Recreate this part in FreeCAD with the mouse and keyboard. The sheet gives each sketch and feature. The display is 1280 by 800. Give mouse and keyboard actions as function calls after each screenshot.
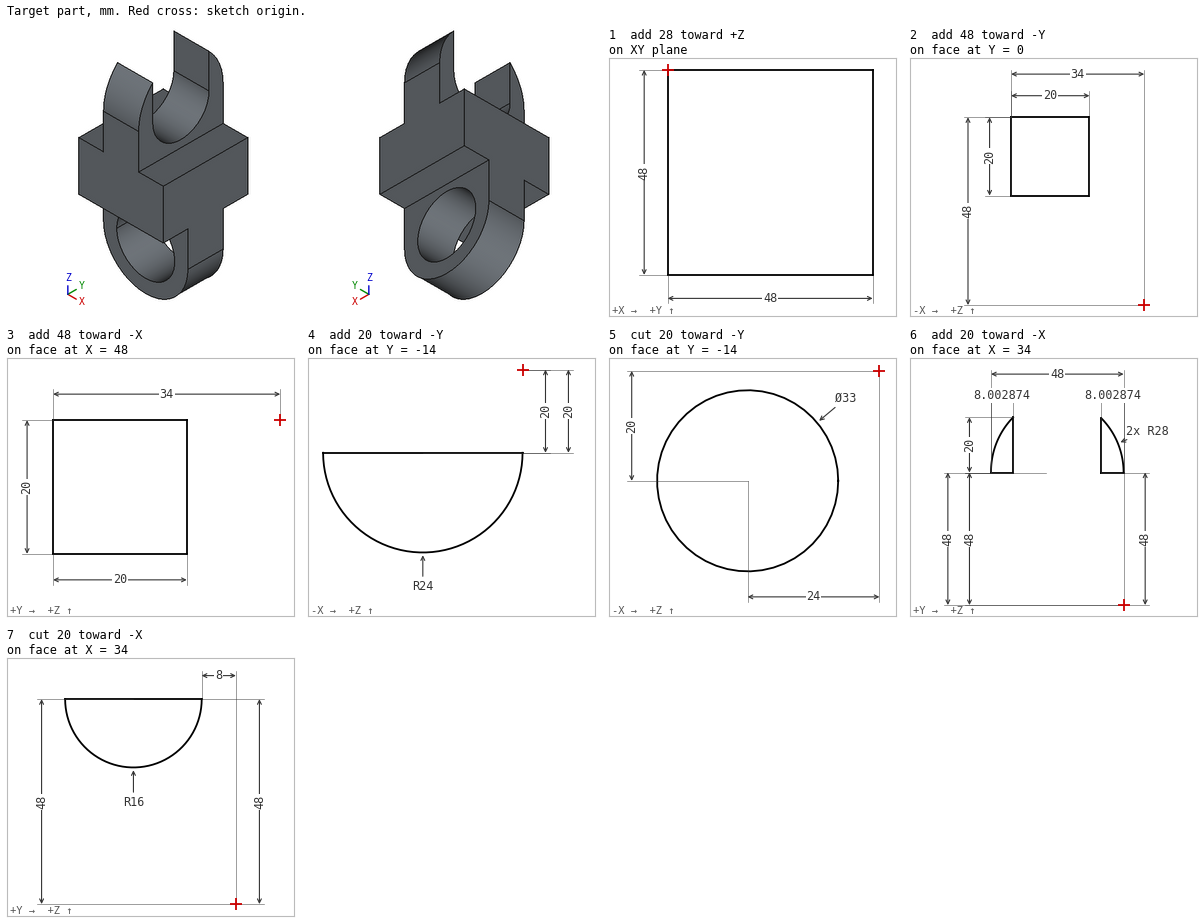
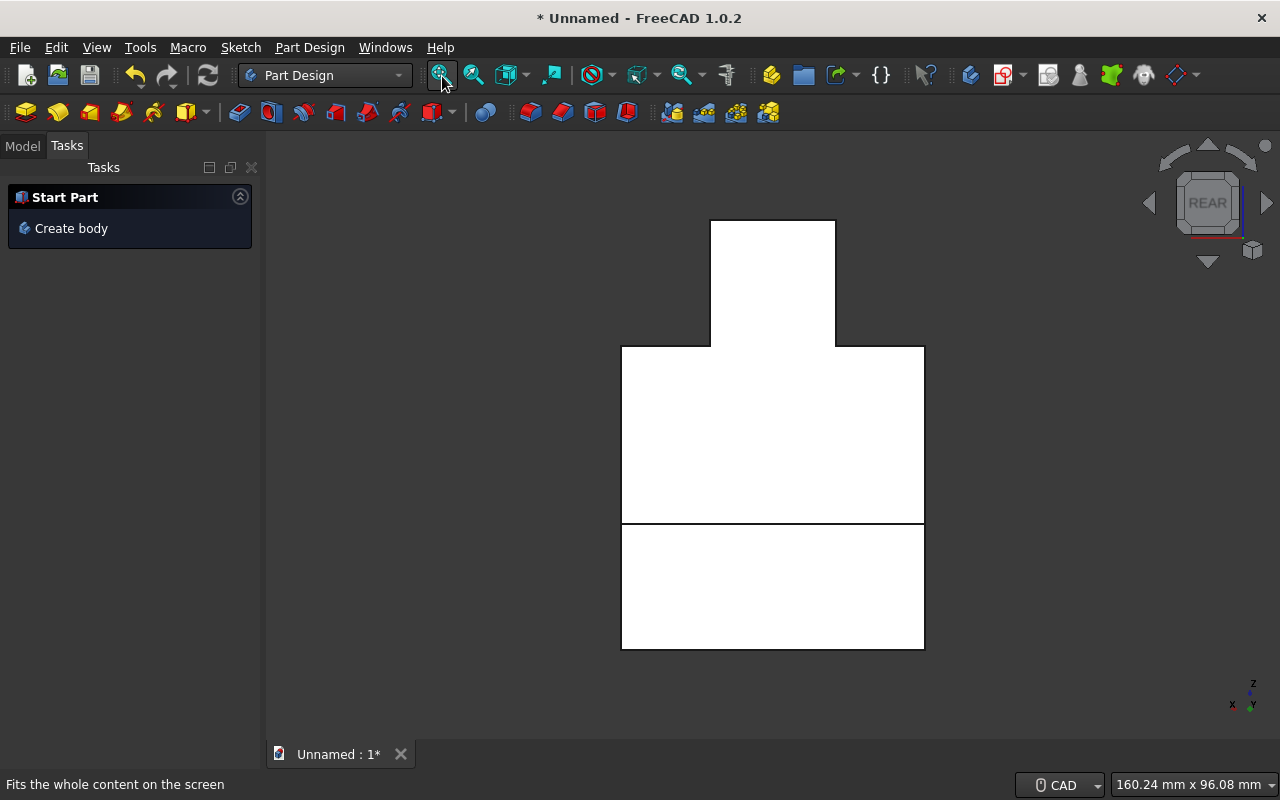
click(686, 586)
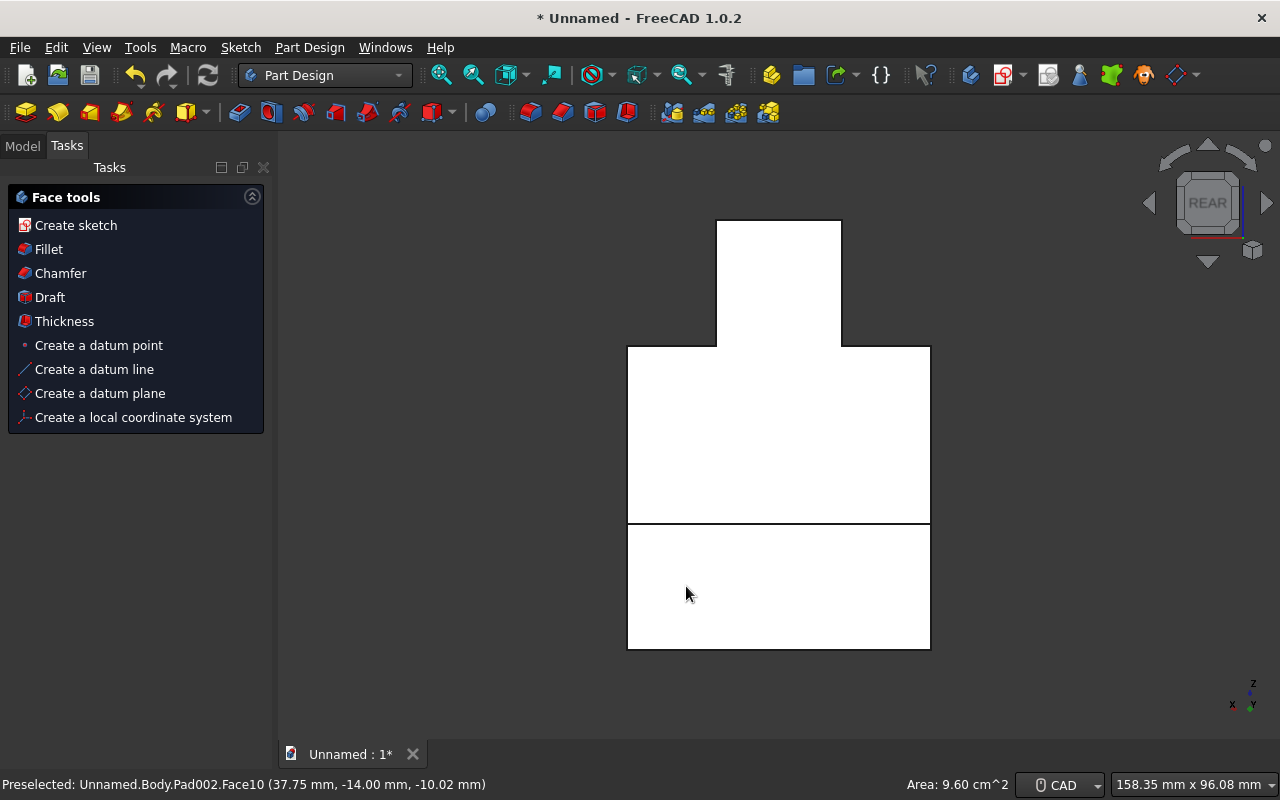
click(1004, 76)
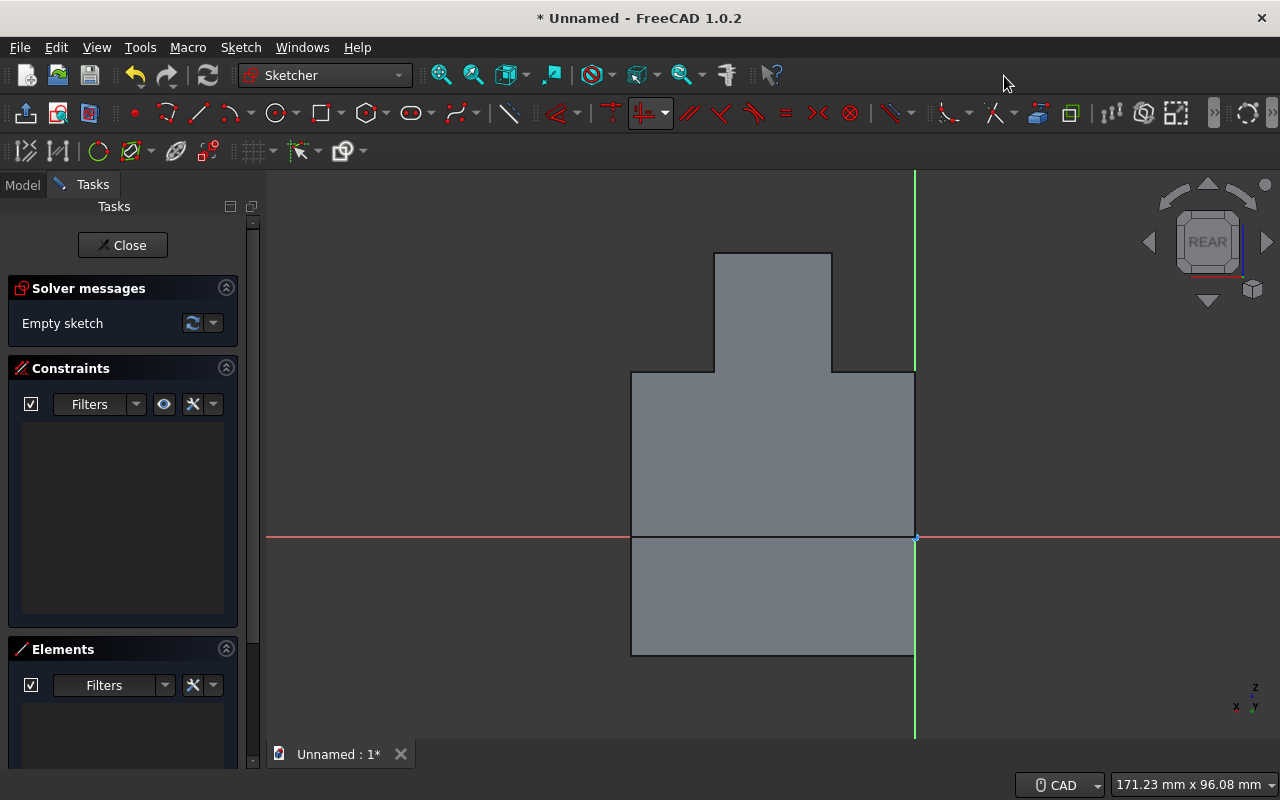
key(q)
key(s)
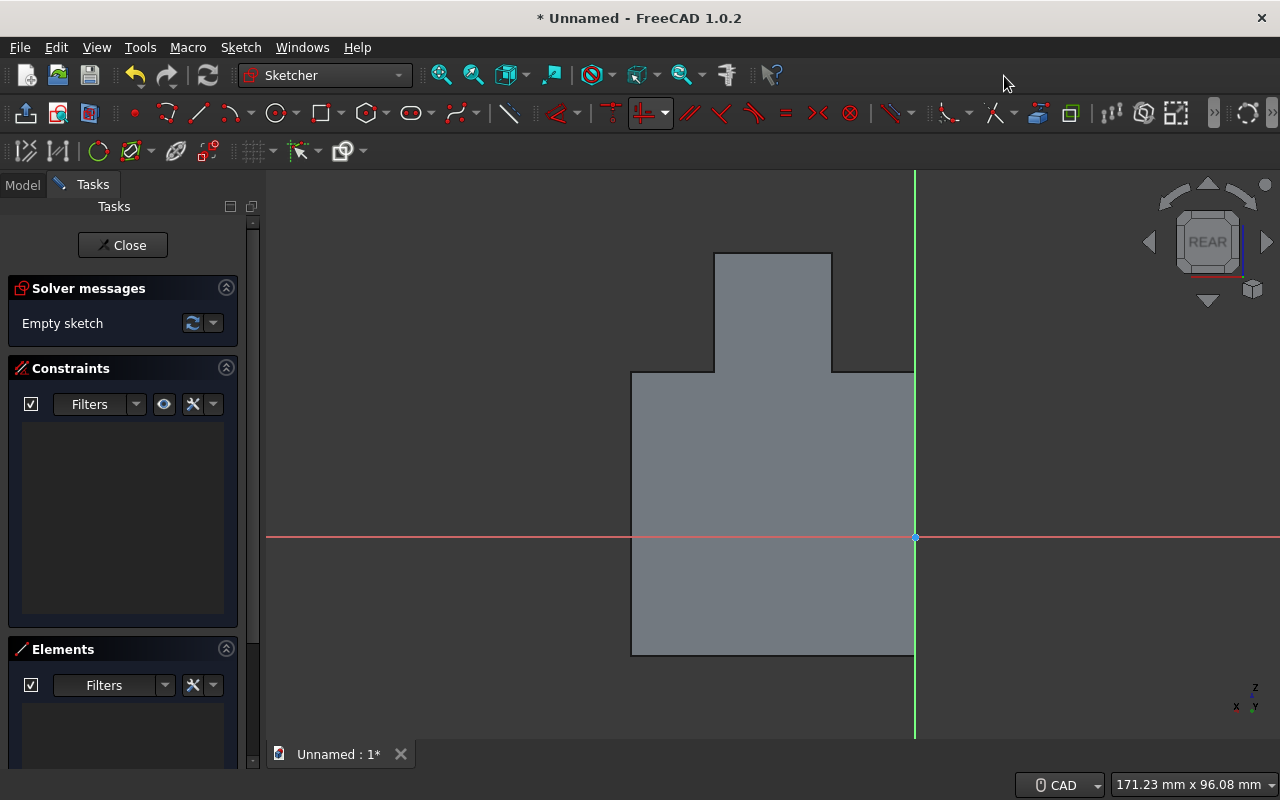
scroll(704, 454, down, 5)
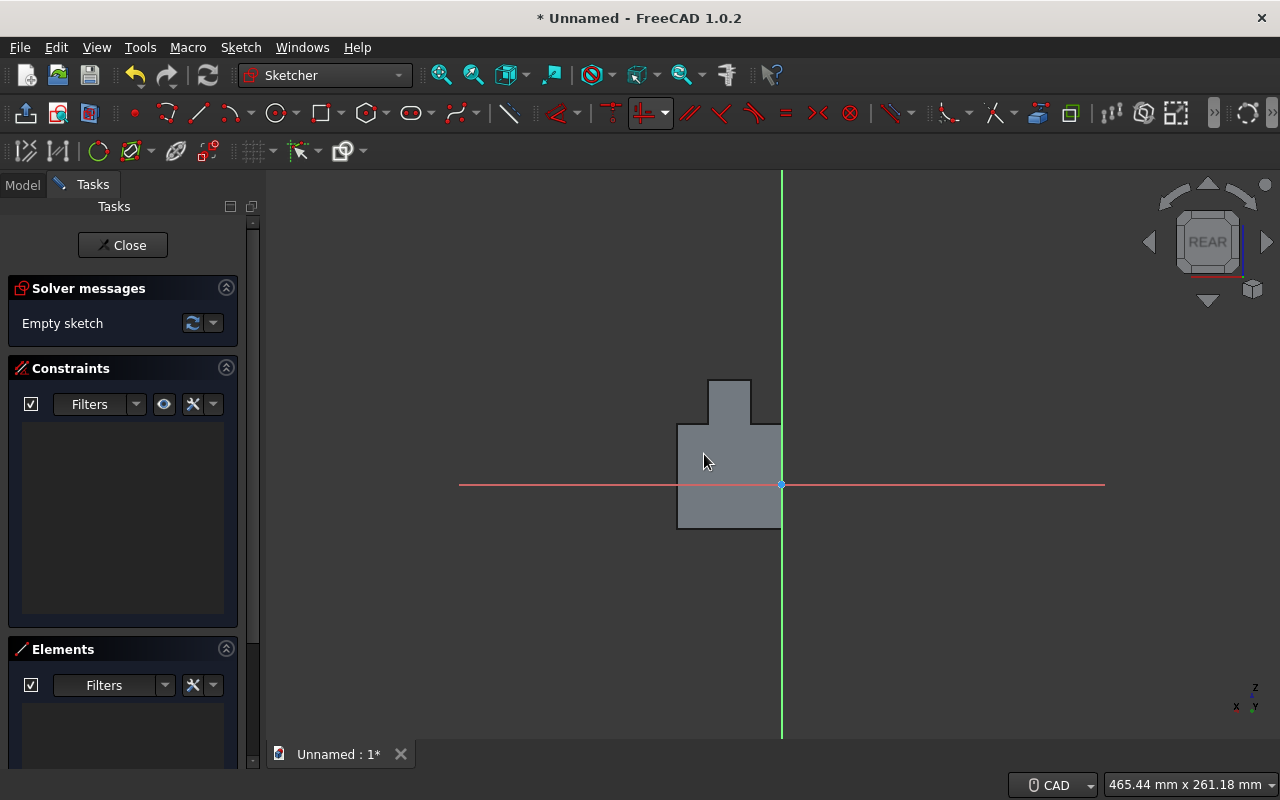
scroll(738, 559, up, 7)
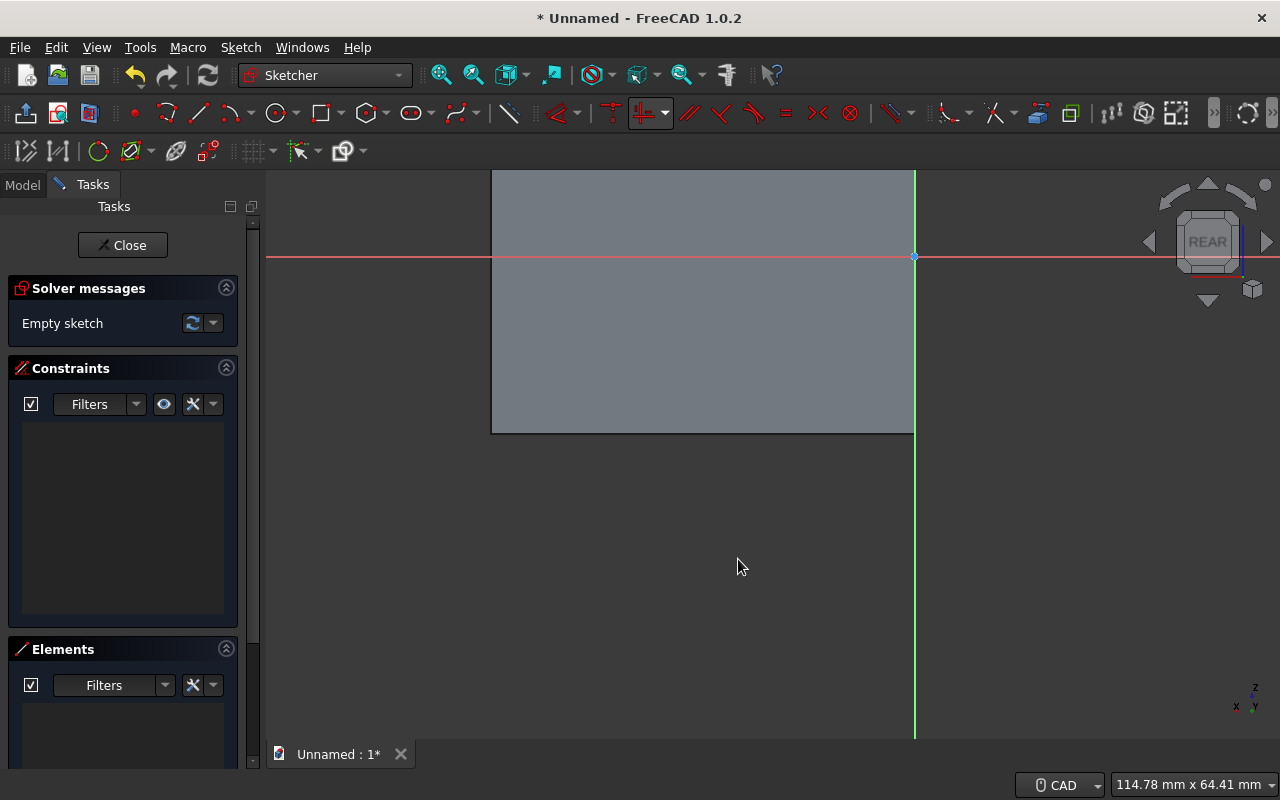
click(200, 114)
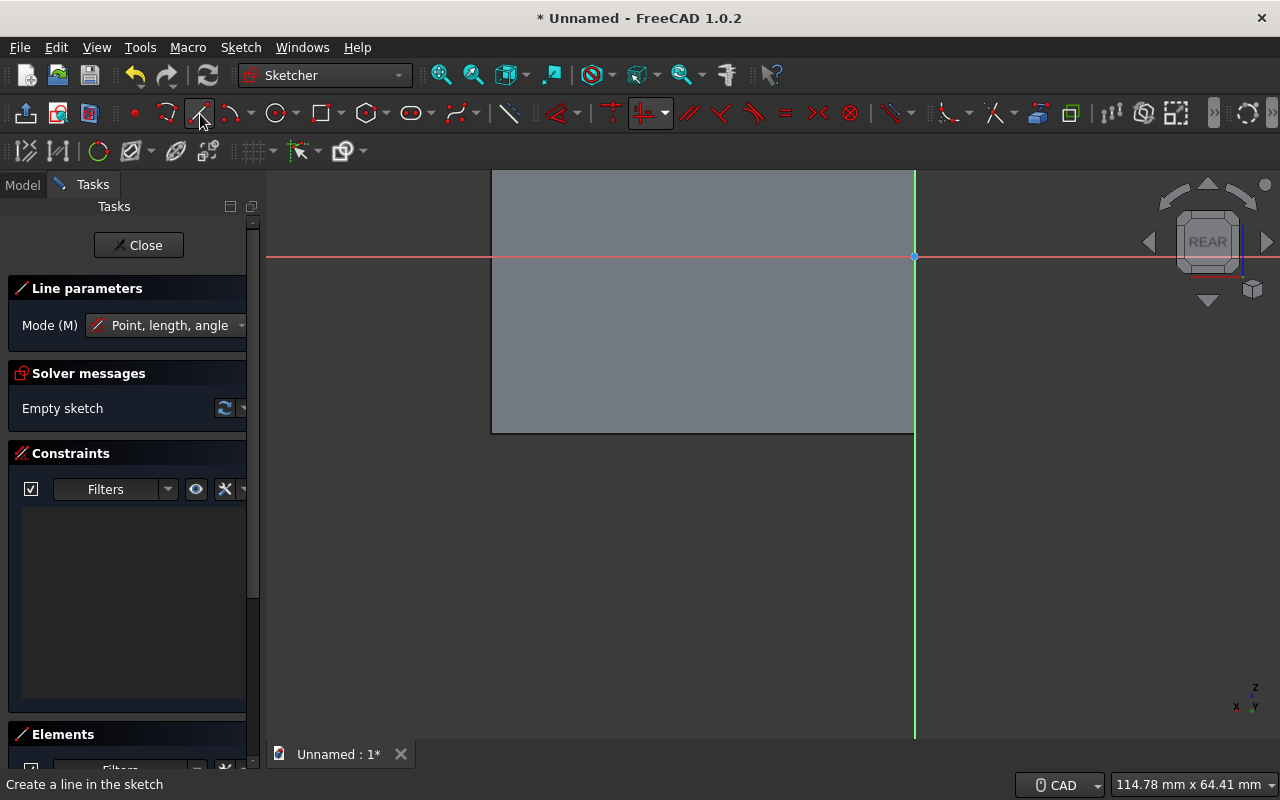
click(915, 434)
click(491, 434)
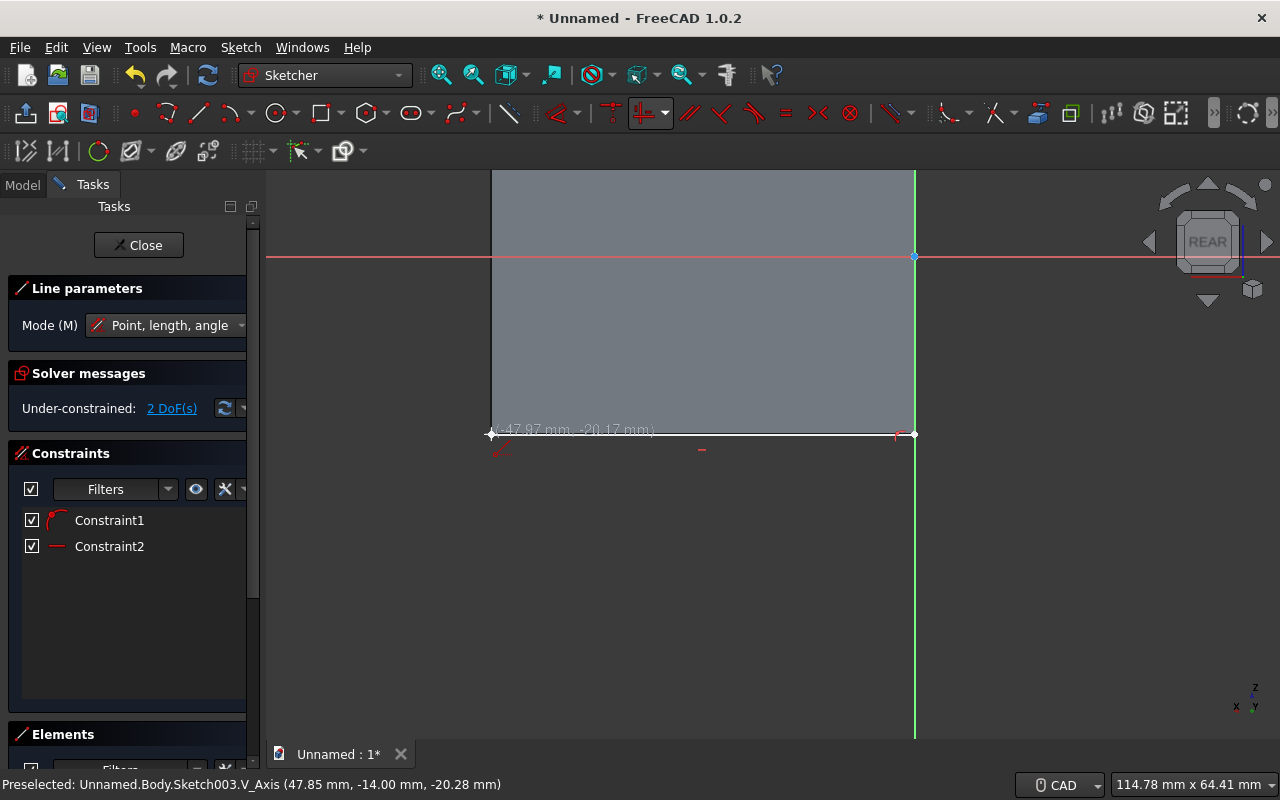
key(g)
key(3)
key(a)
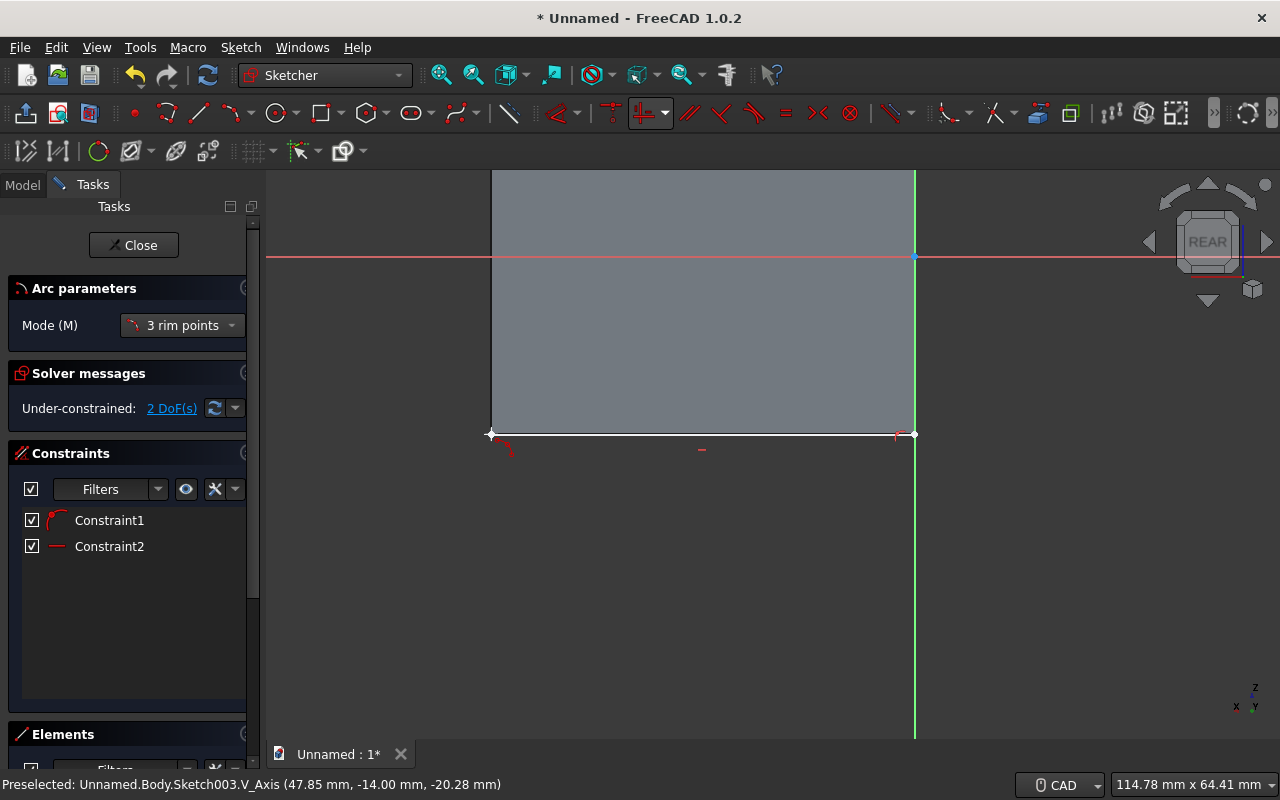
click(491, 435)
click(915, 435)
click(703, 646)
key(Escape)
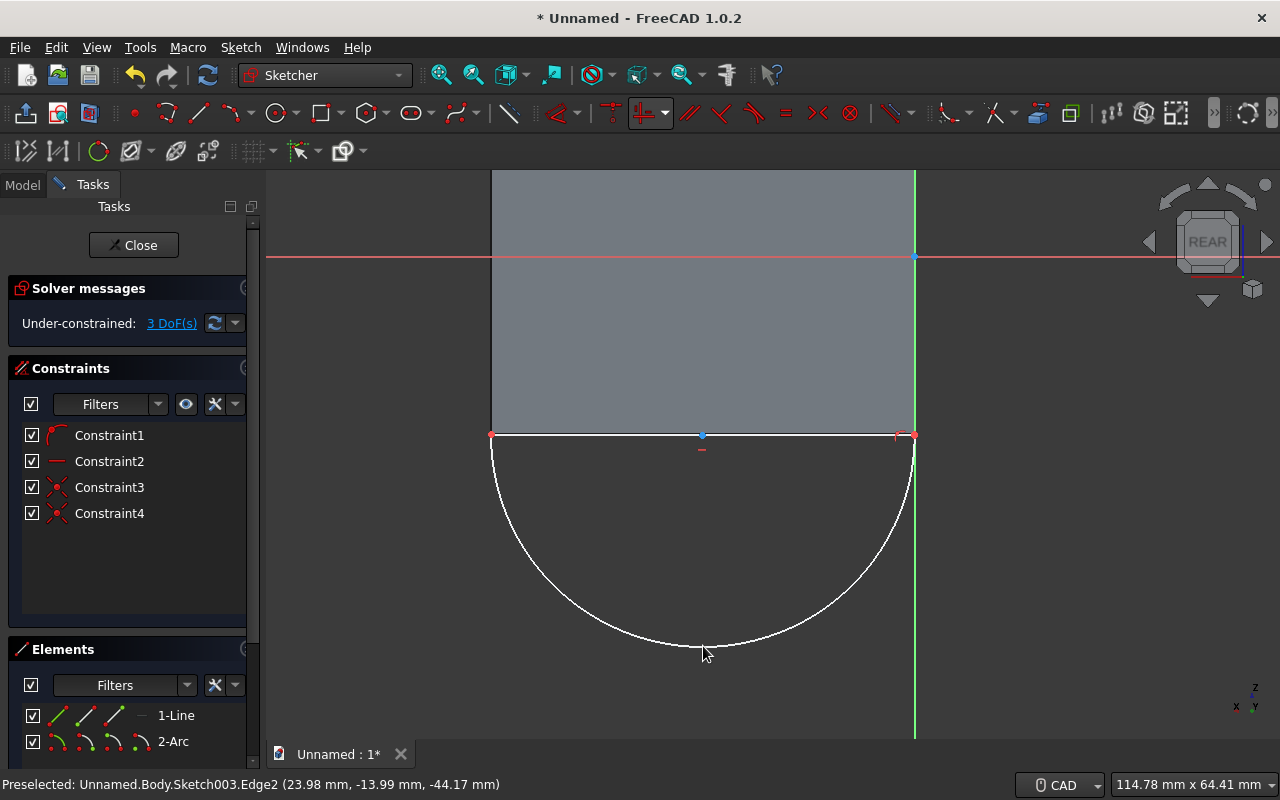
key(d)